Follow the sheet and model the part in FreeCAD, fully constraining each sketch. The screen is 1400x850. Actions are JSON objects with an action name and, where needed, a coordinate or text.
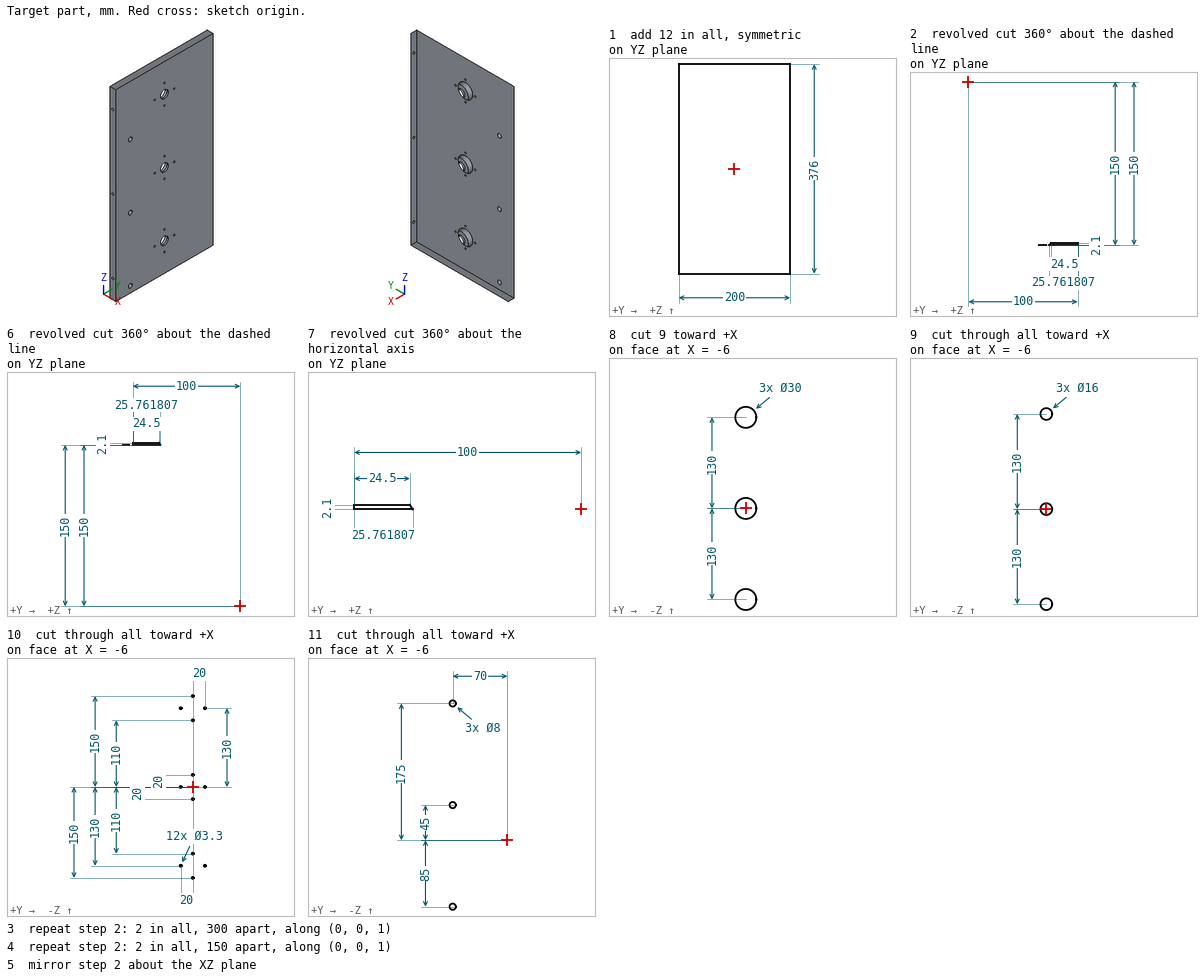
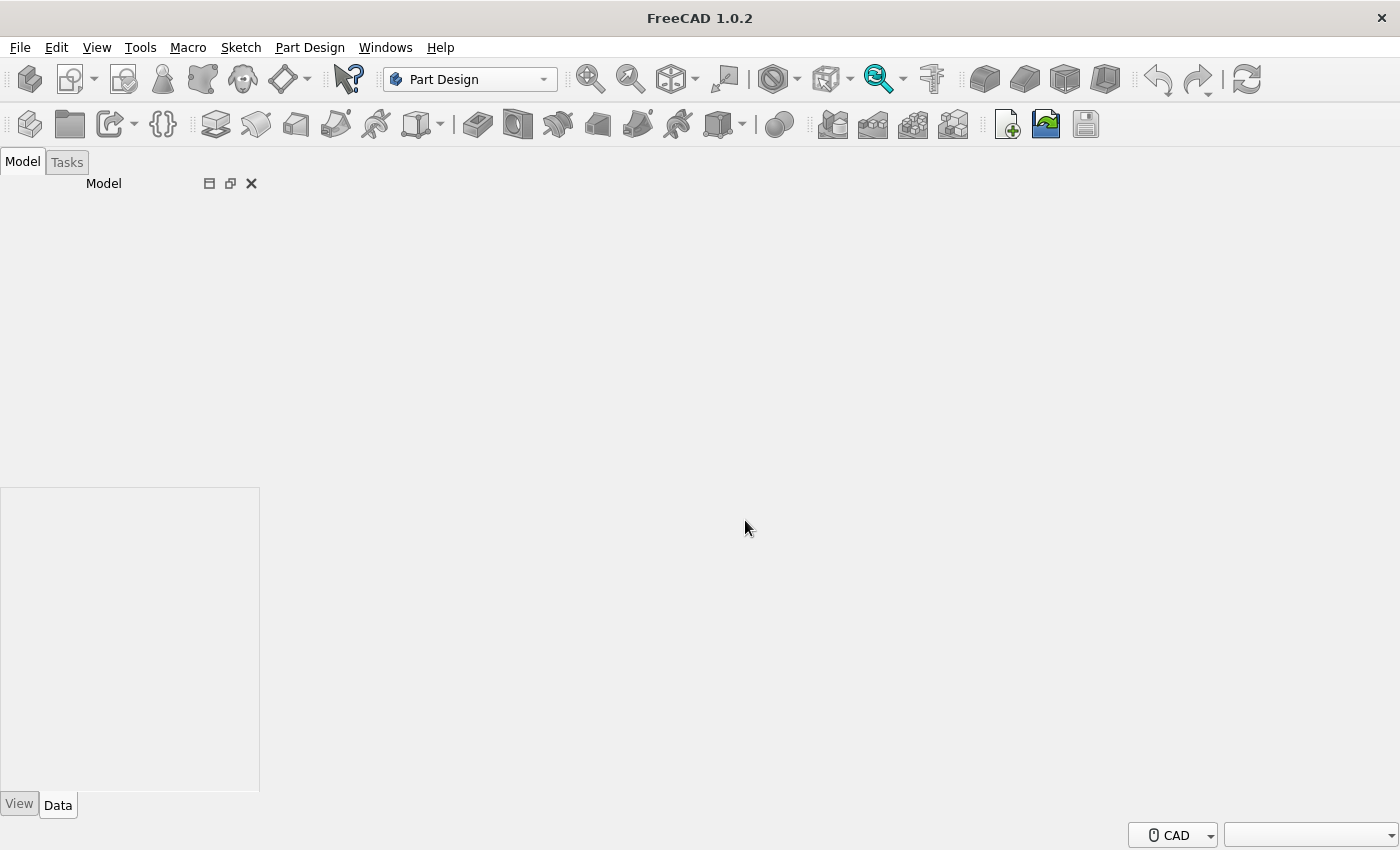
{"action": "left_click", "coordinate": [1006, 124]}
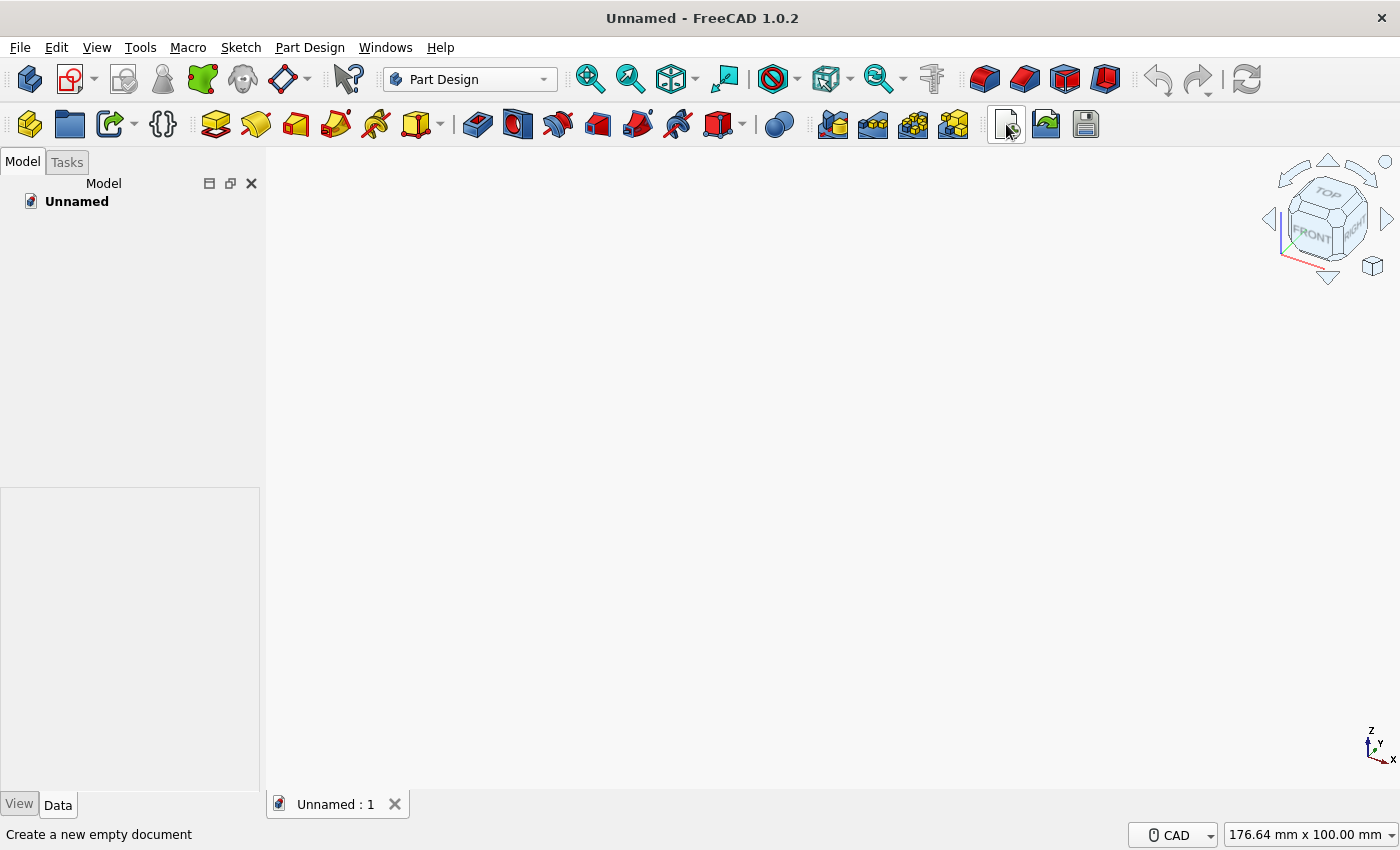
{"action": "left_click", "coordinate": [70, 80]}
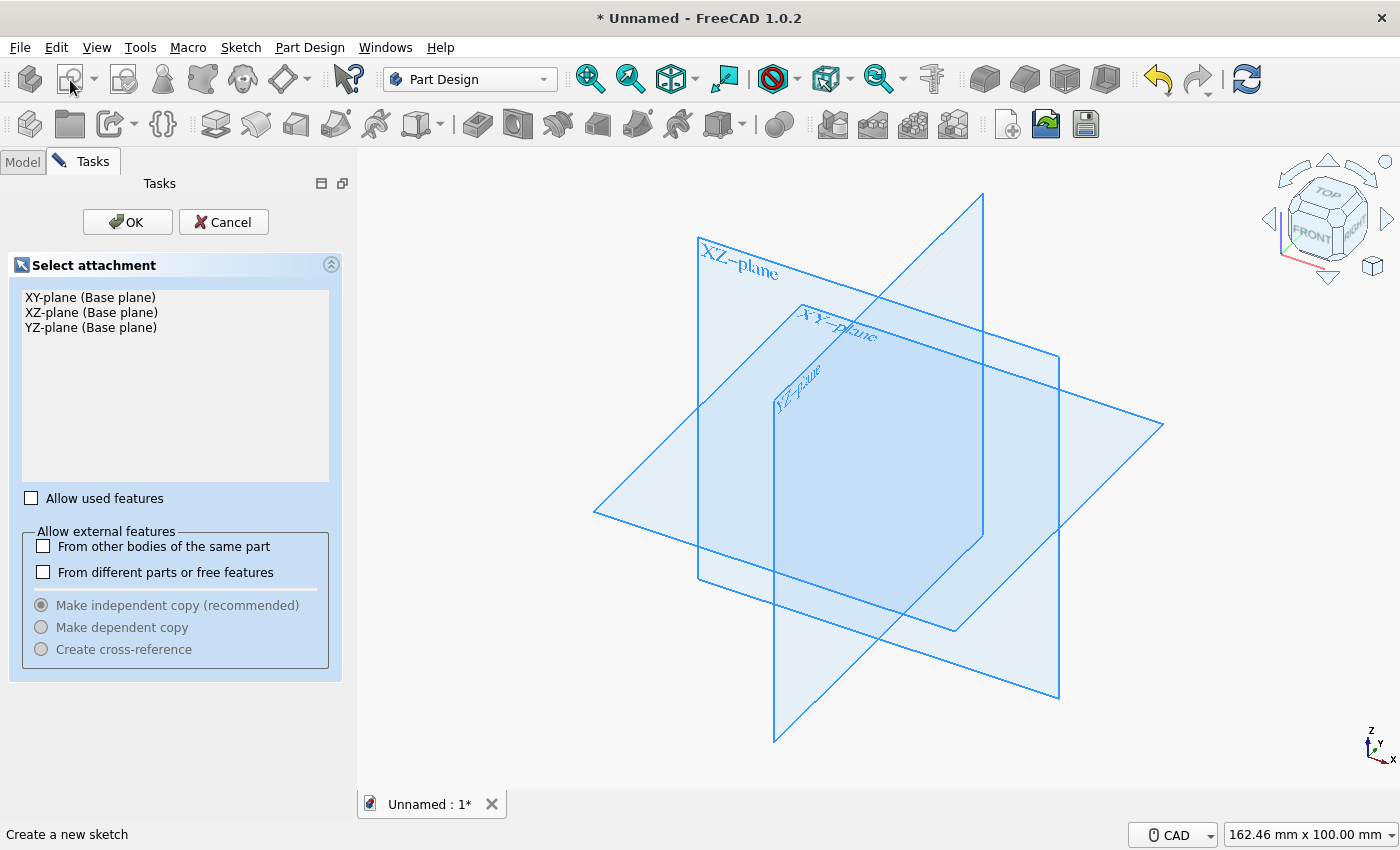
{"action": "left_click", "coordinate": [82, 328]}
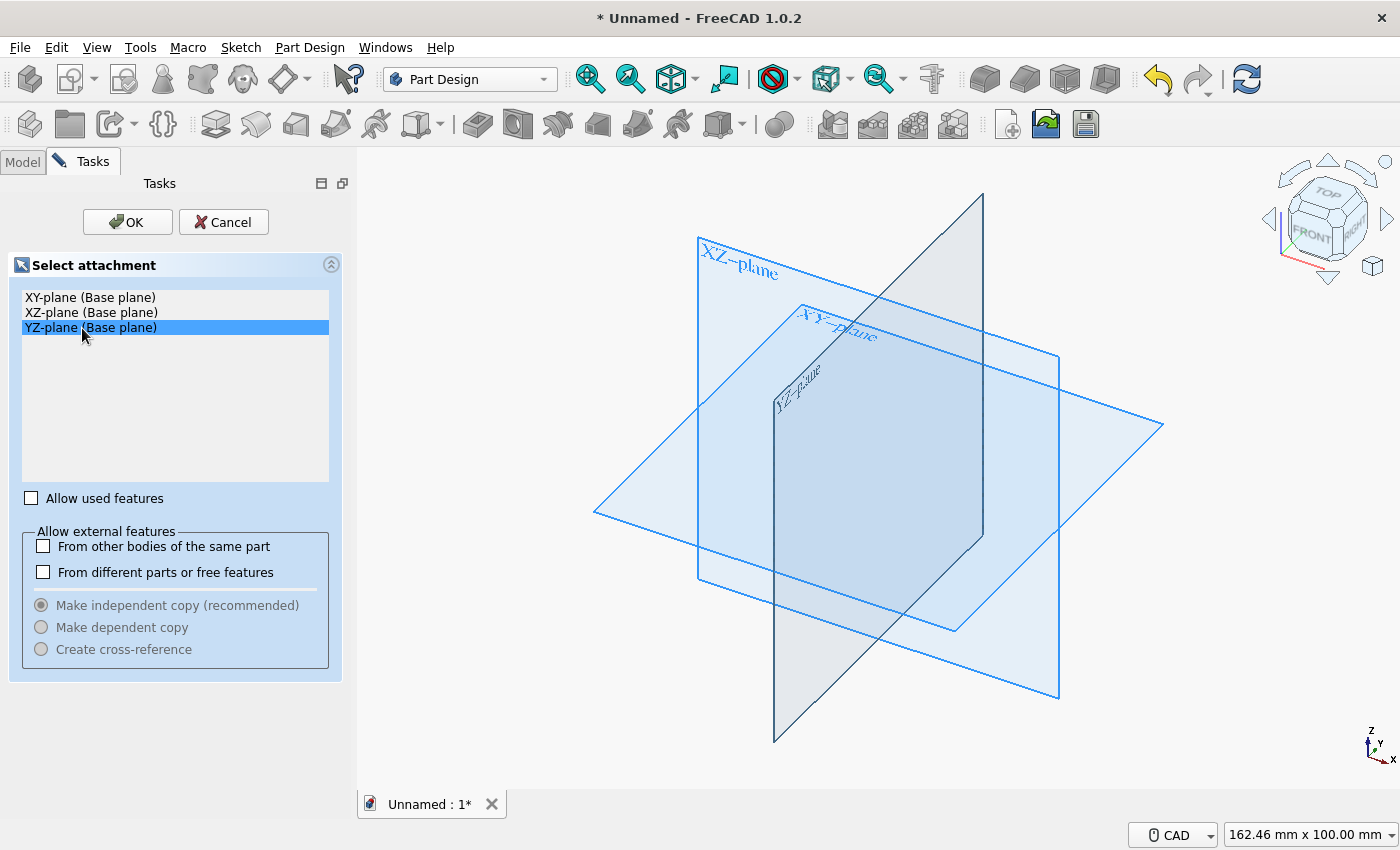
{"action": "left_click", "coordinate": [128, 222]}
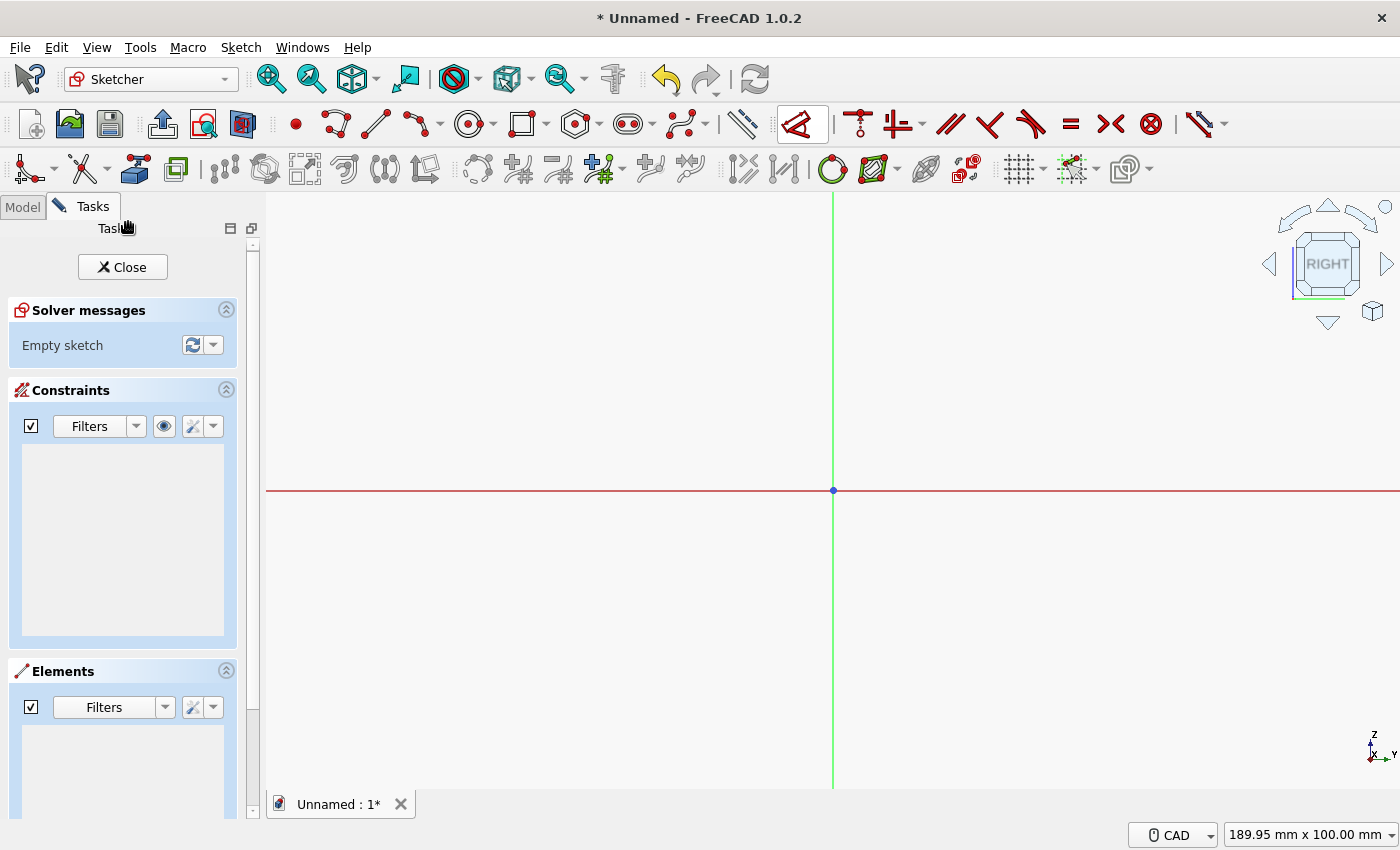
{"action": "scroll", "coordinate": [751, 491], "scroll_direction": "down", "scroll_amount": 9}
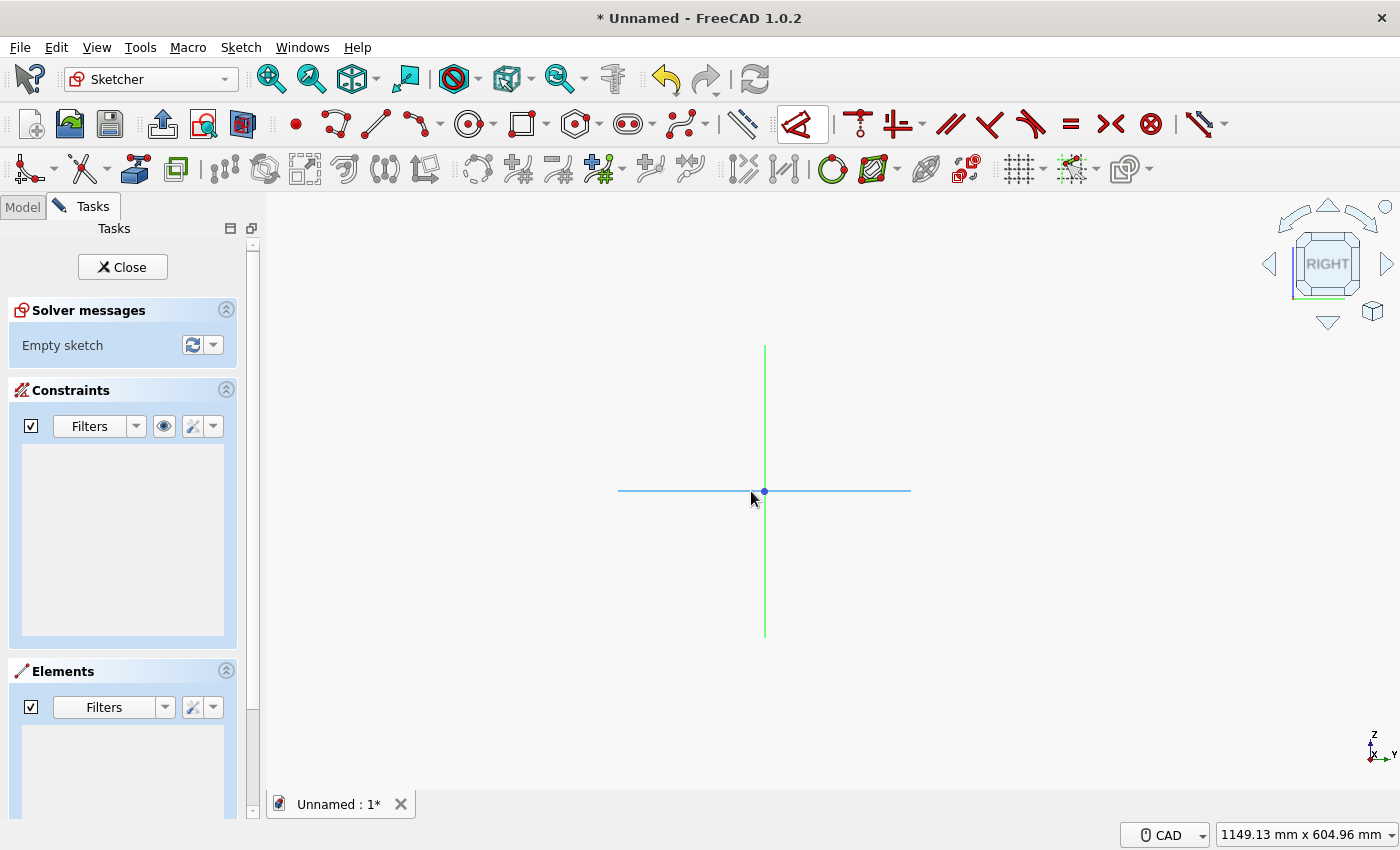
{"action": "left_click", "coordinate": [548, 124]}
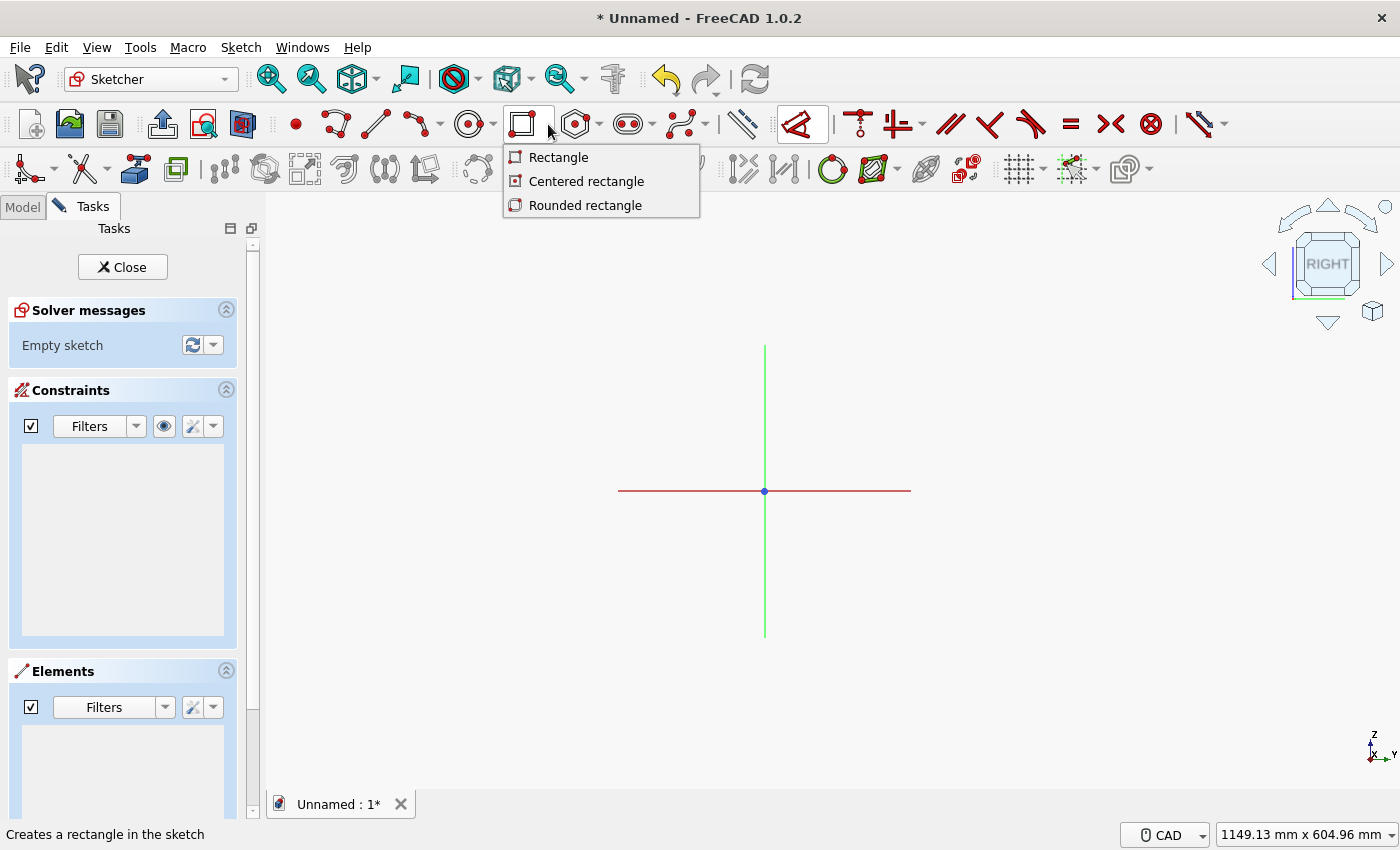
{"action": "left_click", "coordinate": [602, 181]}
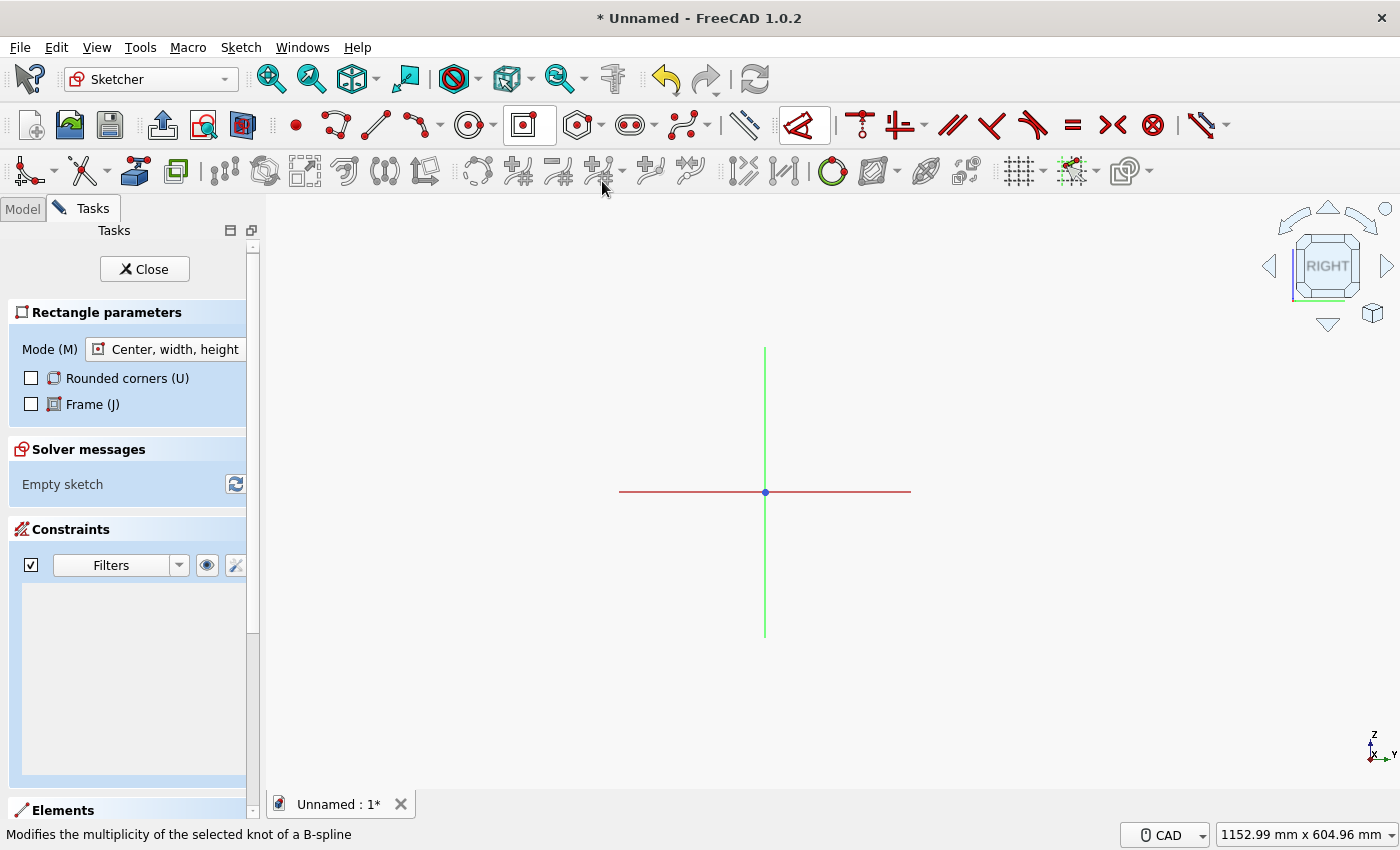
{"action": "left_click", "coordinate": [765, 492]}
{"action": "mouse_move", "coordinate": [863, 307]}